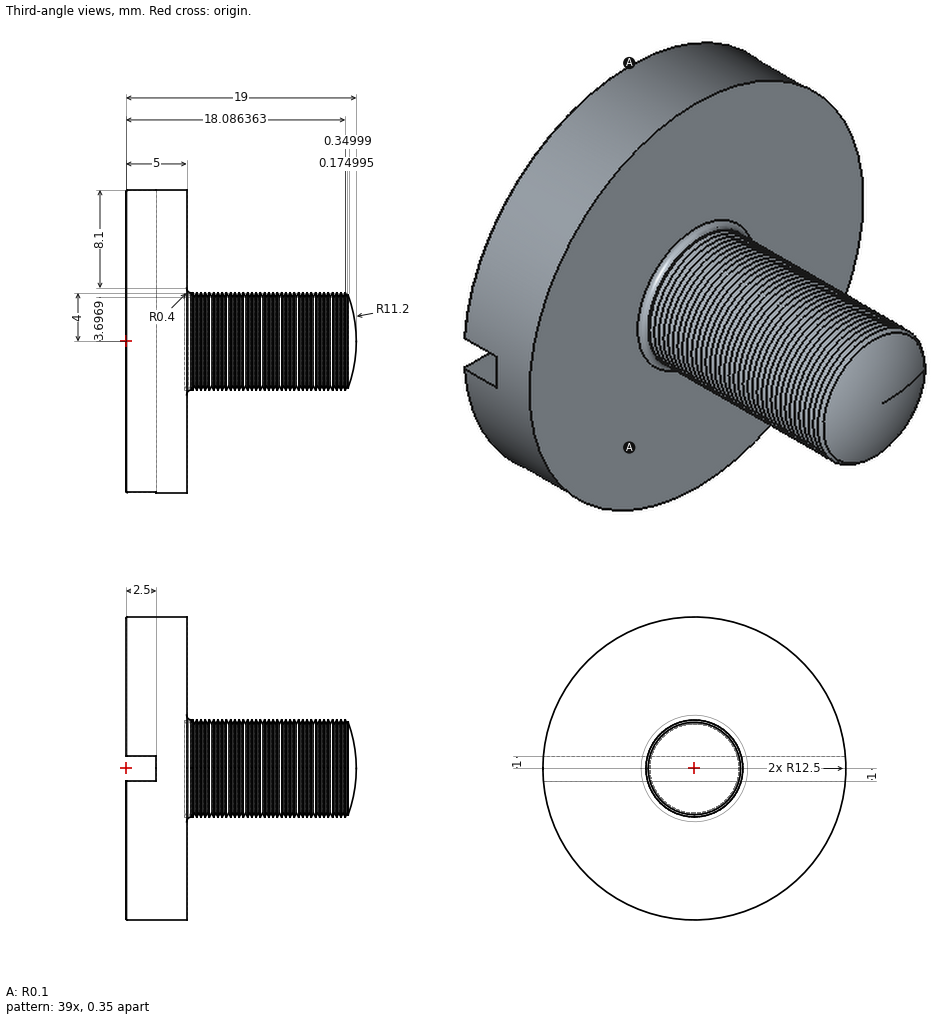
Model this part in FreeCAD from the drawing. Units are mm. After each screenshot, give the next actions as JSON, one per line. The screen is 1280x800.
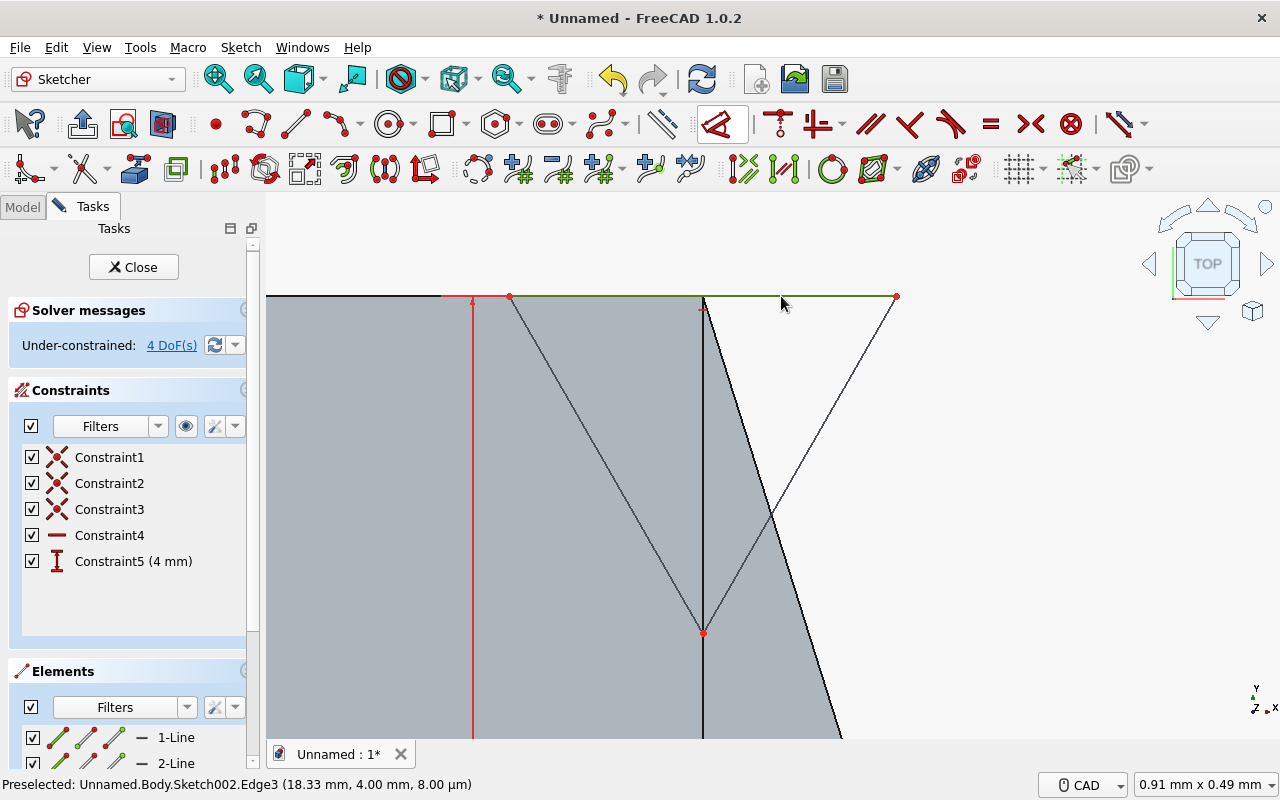
{"action": "left_click", "coordinate": [742, 124]}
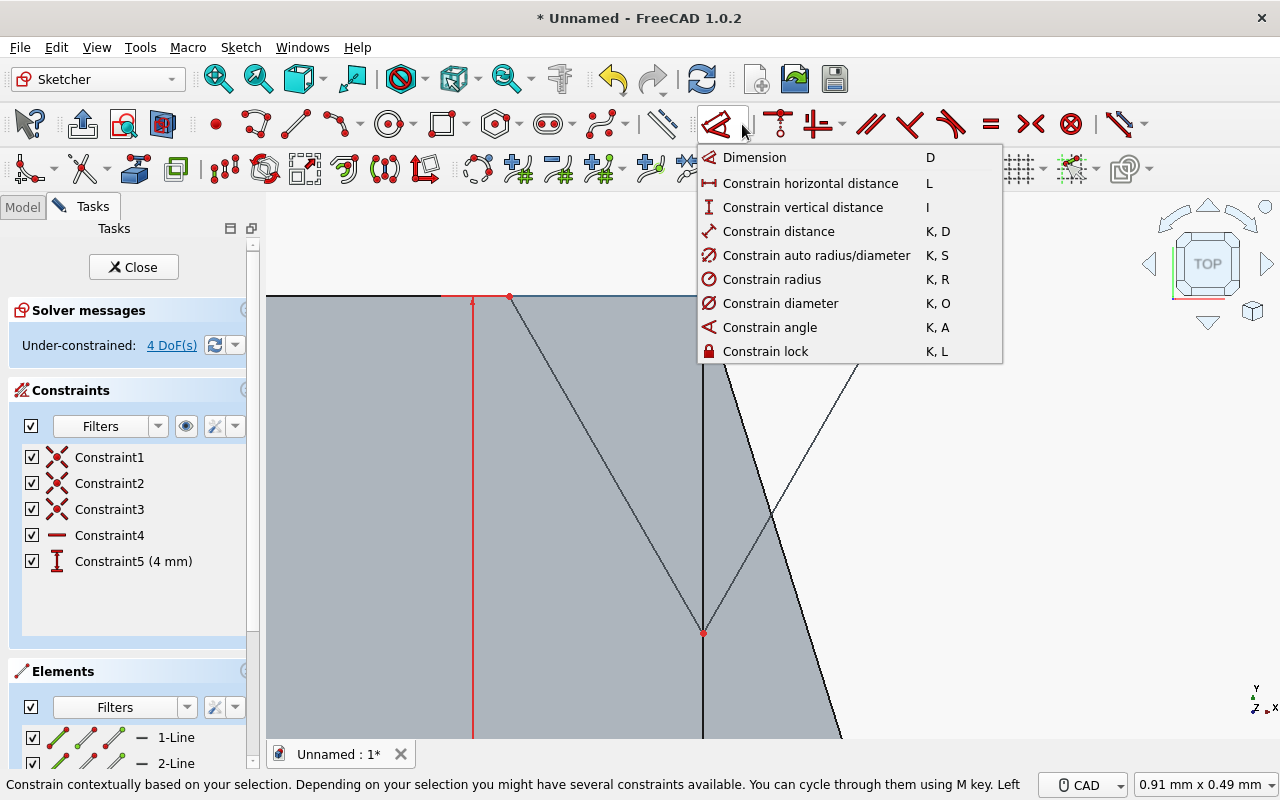
{"action": "left_click", "coordinate": [850, 183]}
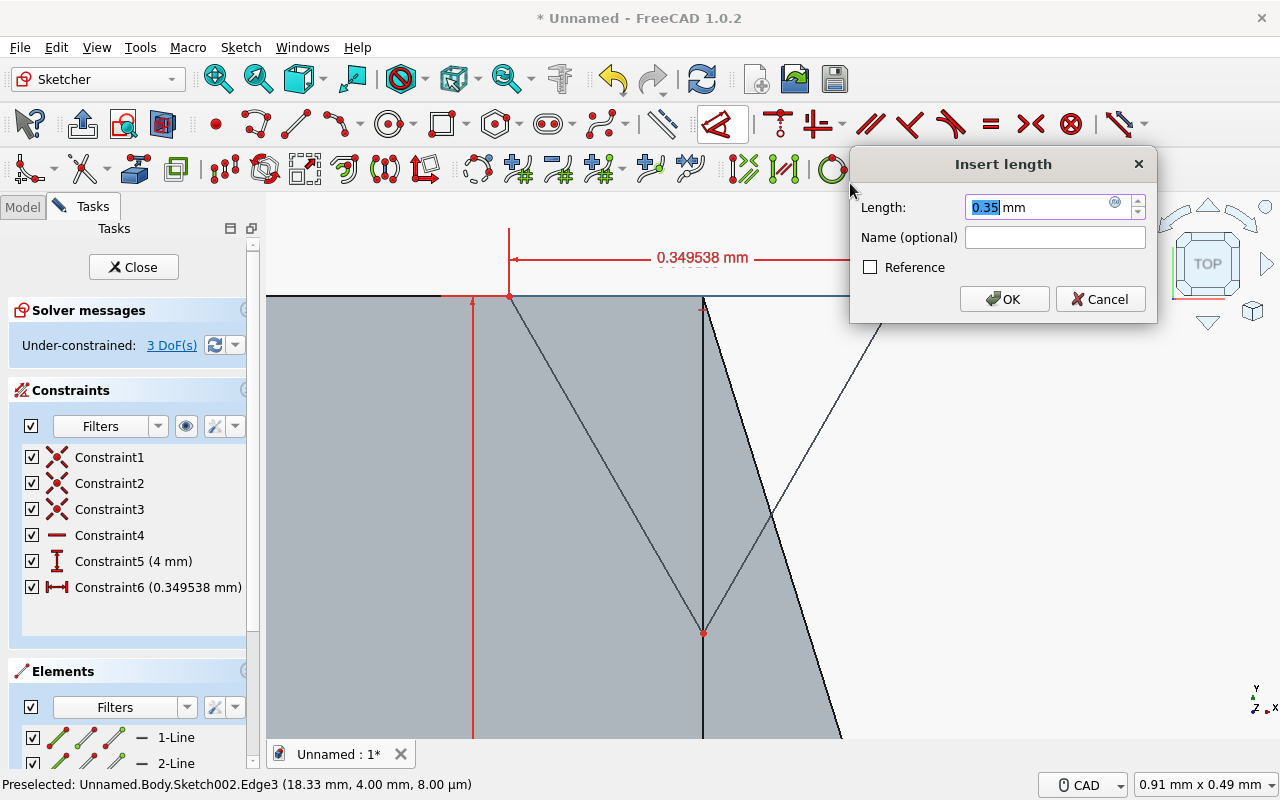
{"action": "type", "text": "0.34999"}
{"action": "key", "text": "Return"}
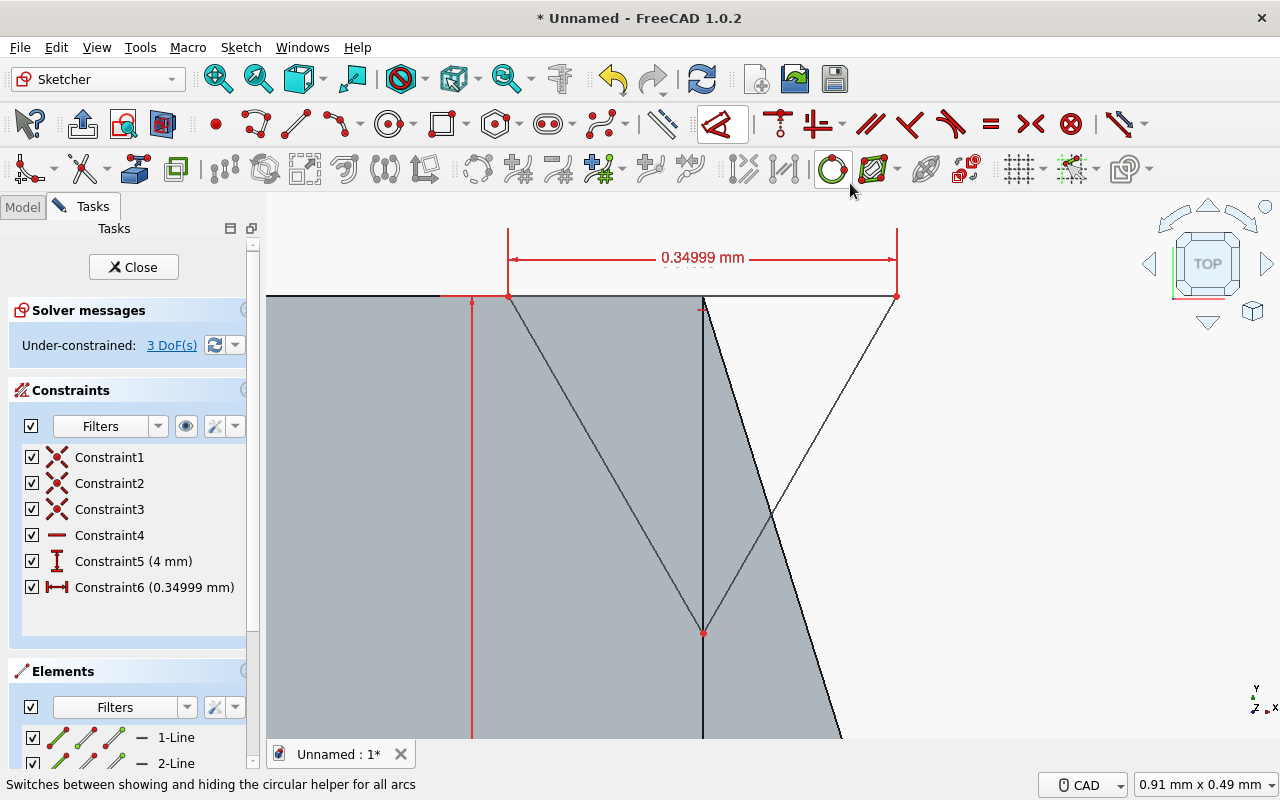
{"action": "left_click", "coordinate": [703, 634]}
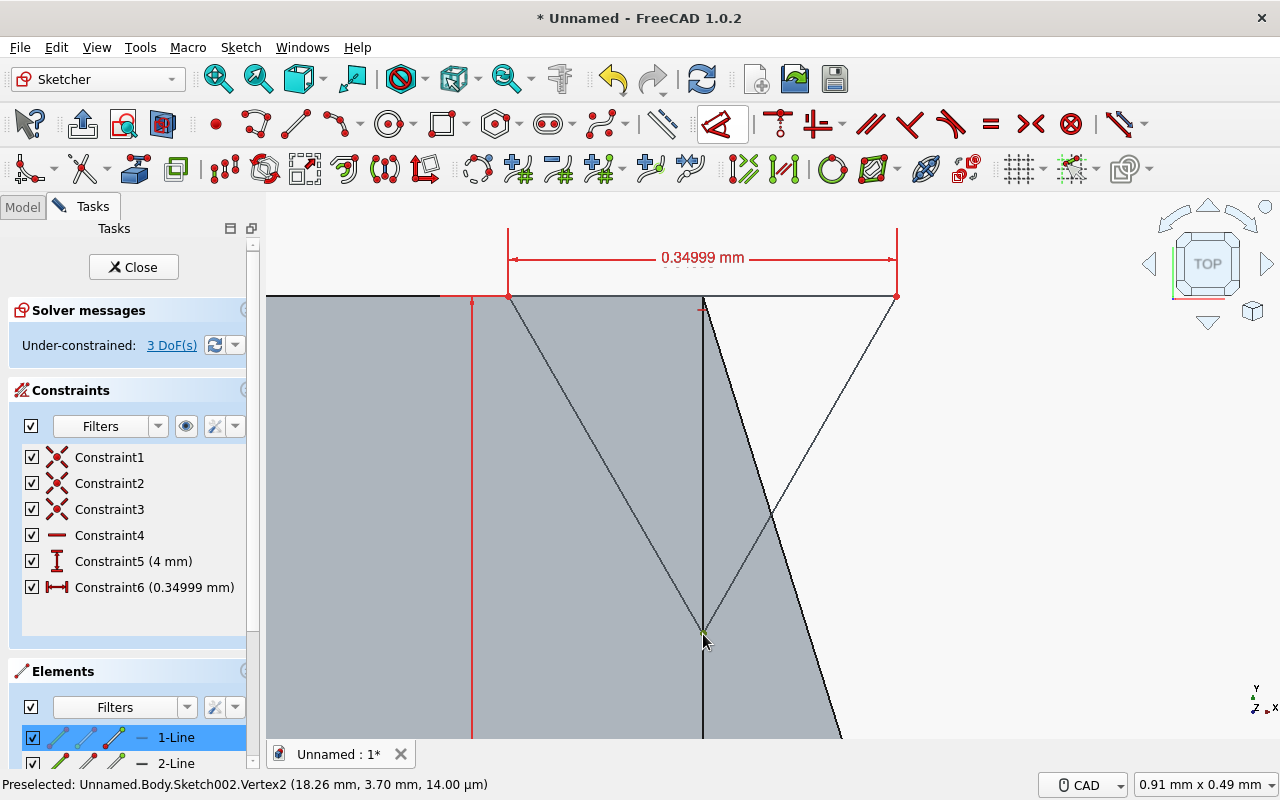
{"action": "left_click", "coordinate": [742, 124]}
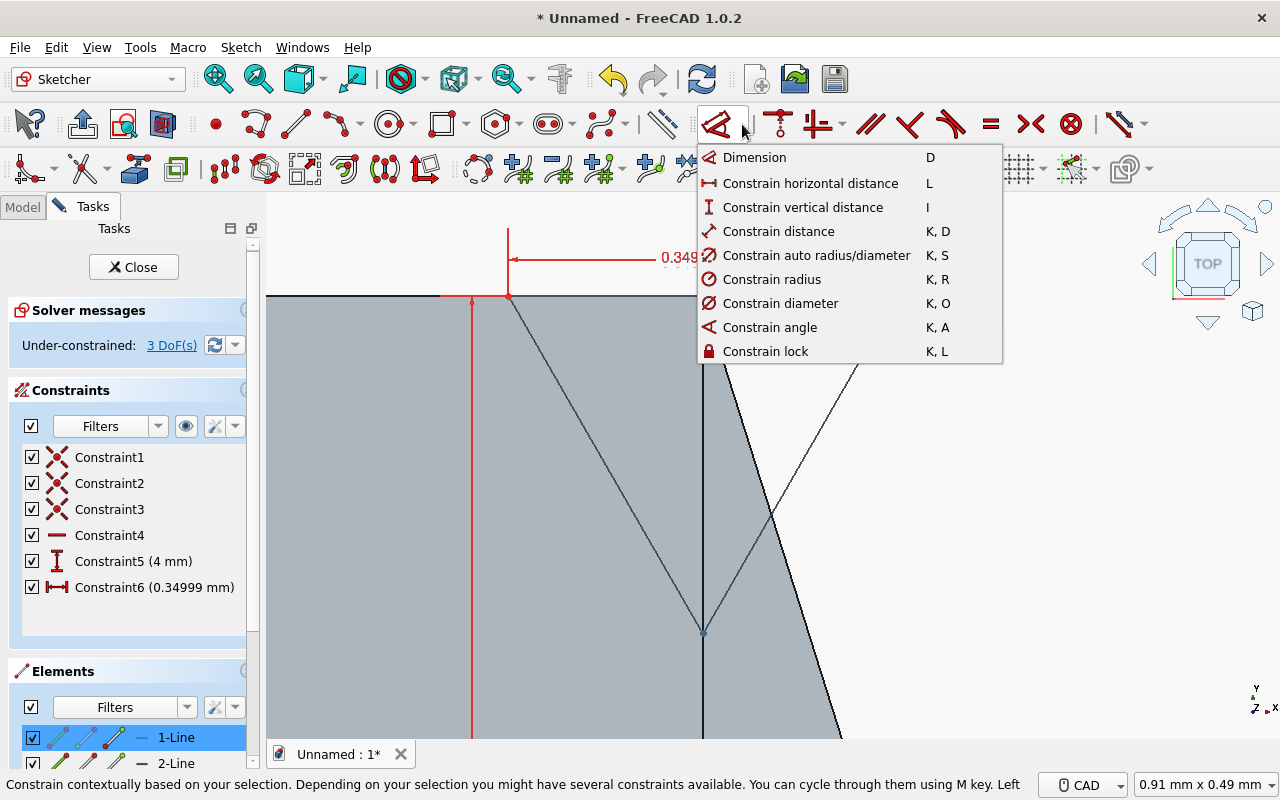
{"action": "left_click", "coordinate": [850, 207]}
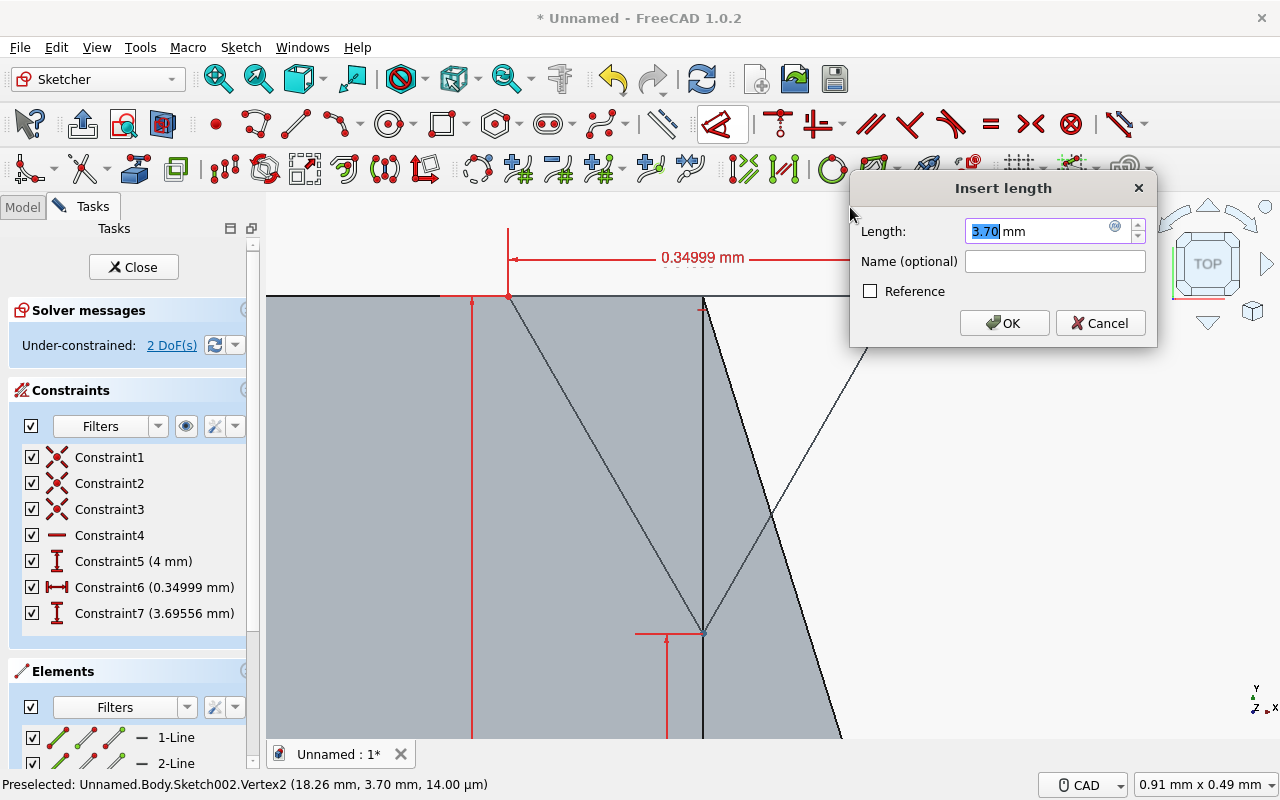
{"action": "type", "text": "3.6969"}
{"action": "key", "text": "Return"}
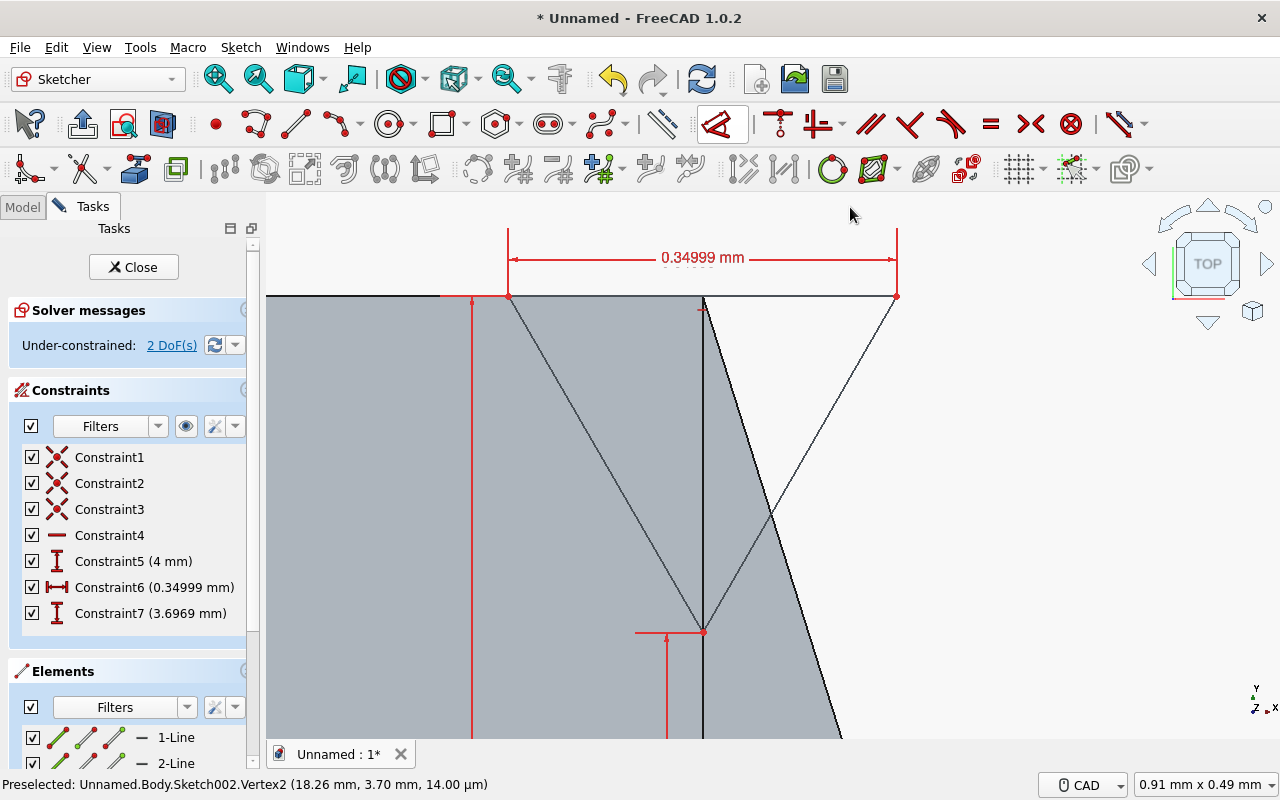
{"action": "left_click", "coordinate": [567, 397]}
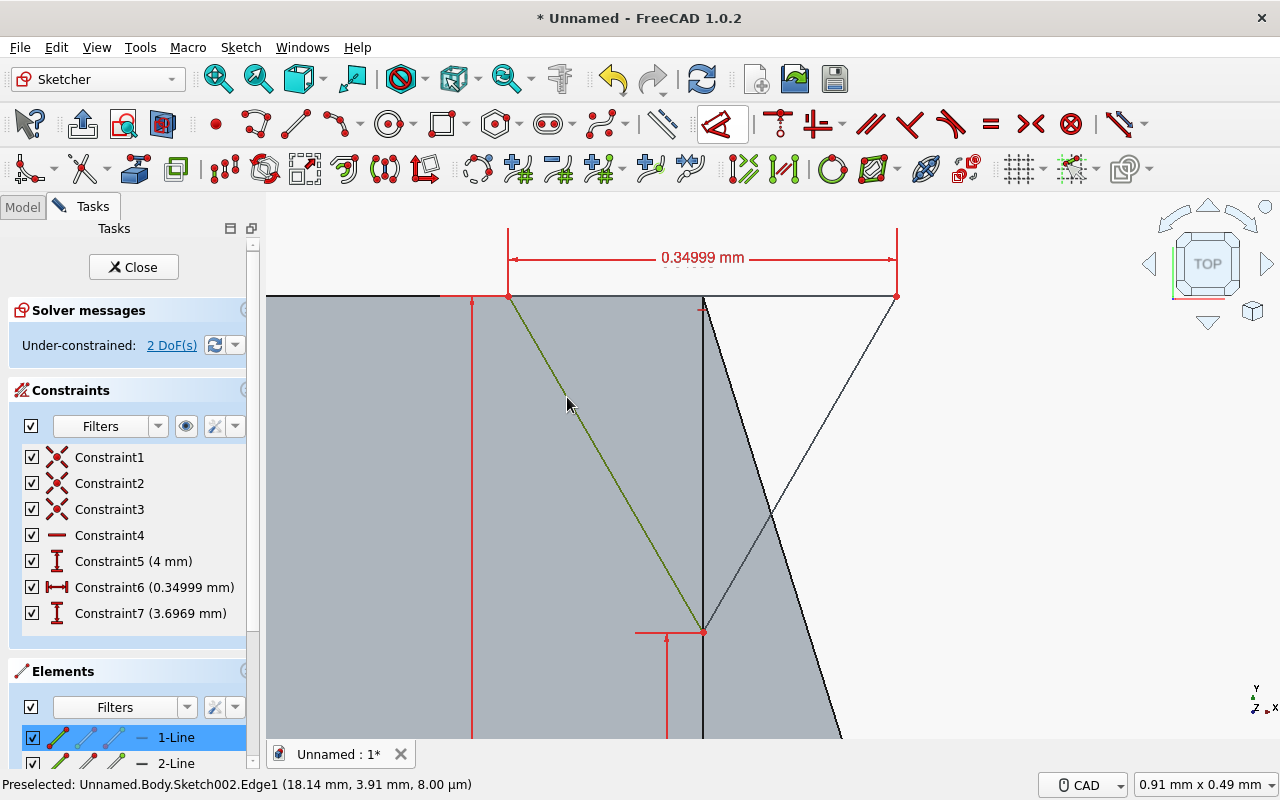
{"action": "left_click", "coordinate": [742, 124]}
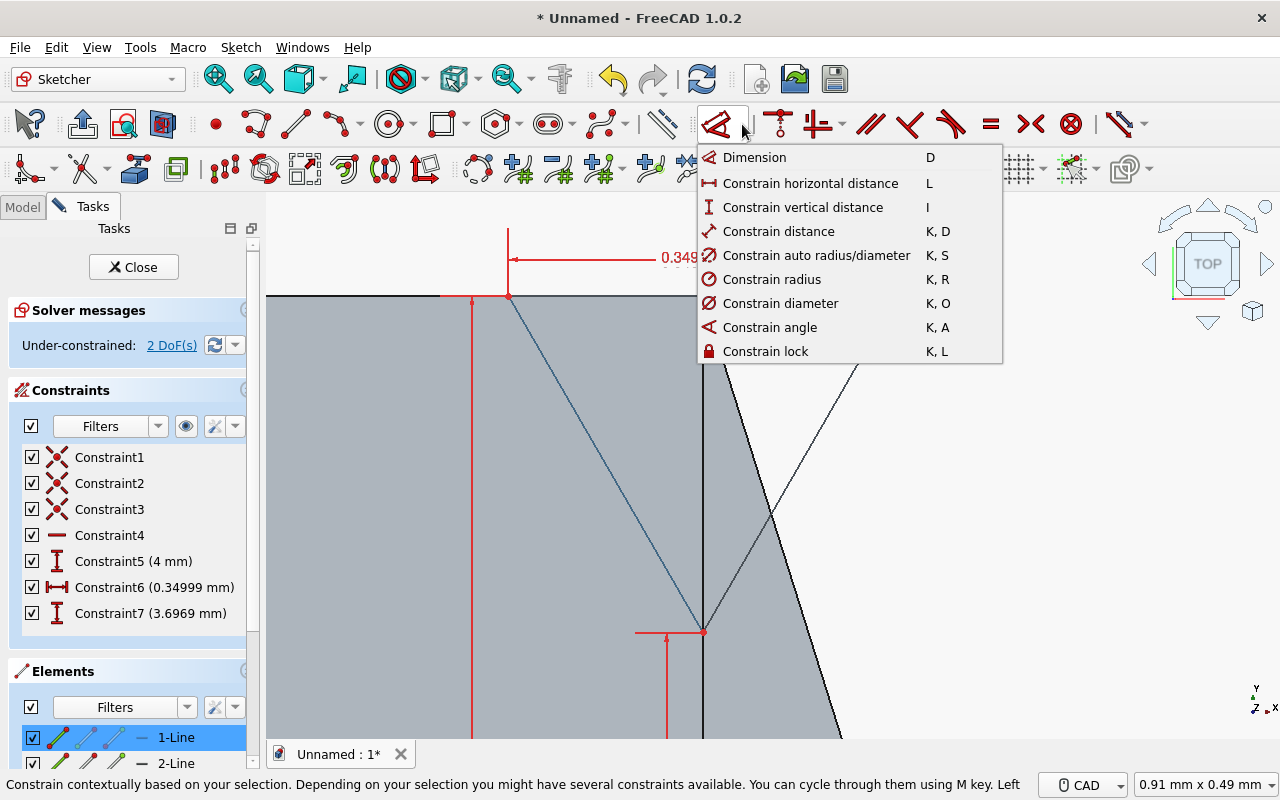
{"action": "left_click", "coordinate": [850, 183]}